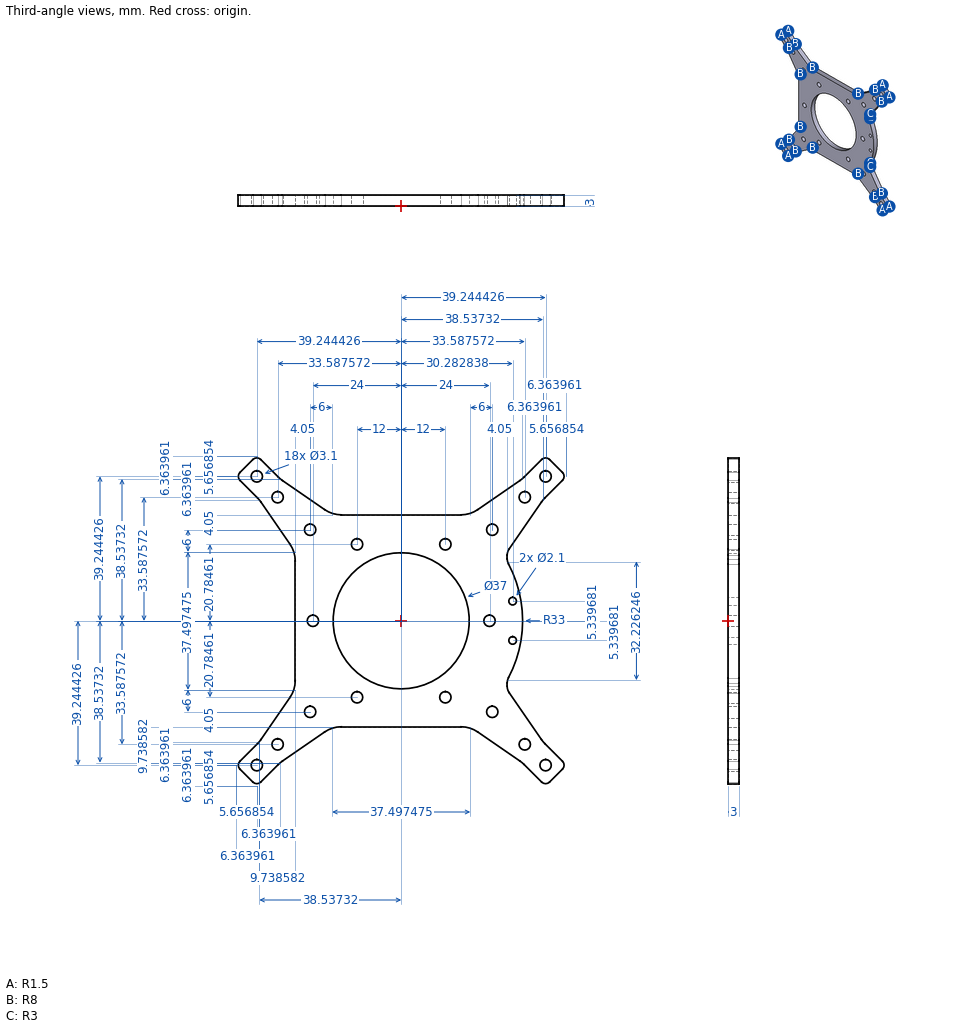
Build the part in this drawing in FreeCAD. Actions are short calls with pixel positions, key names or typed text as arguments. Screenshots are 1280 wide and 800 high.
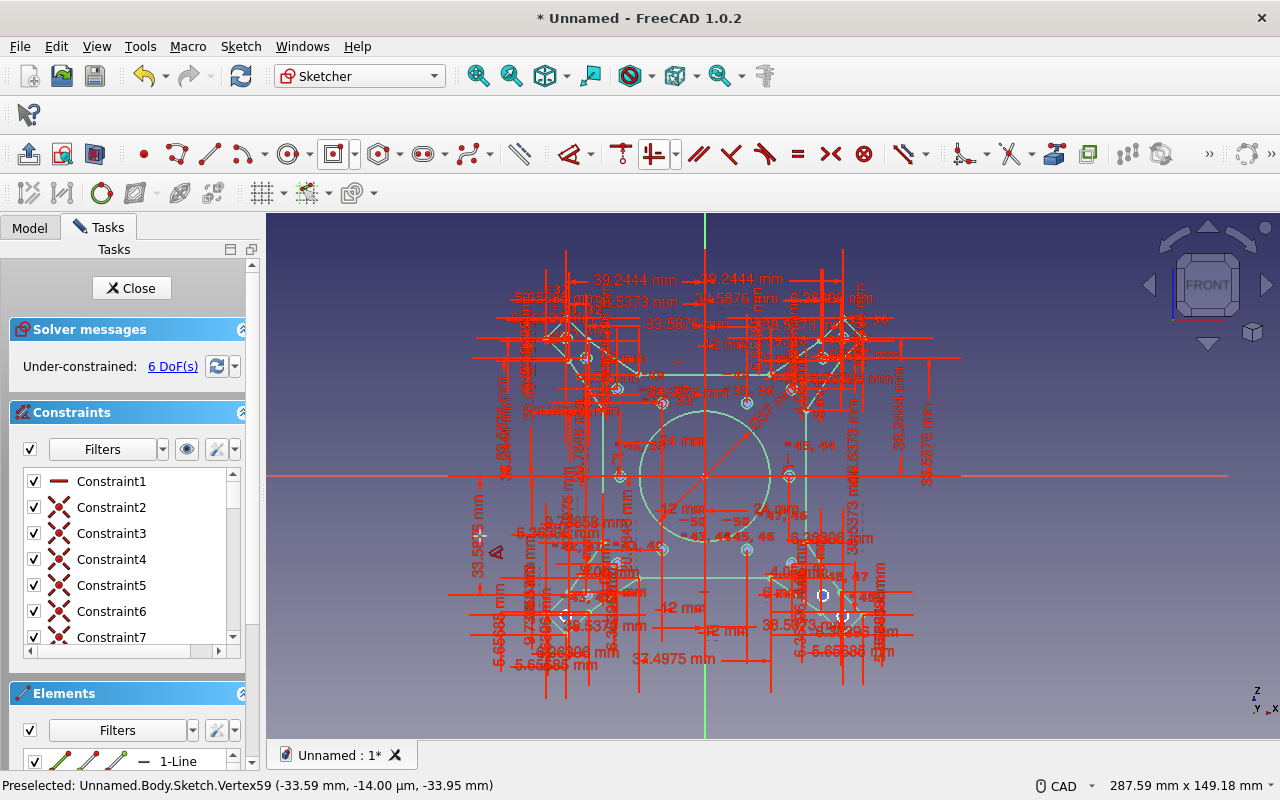
click(566, 616)
click(635, 698)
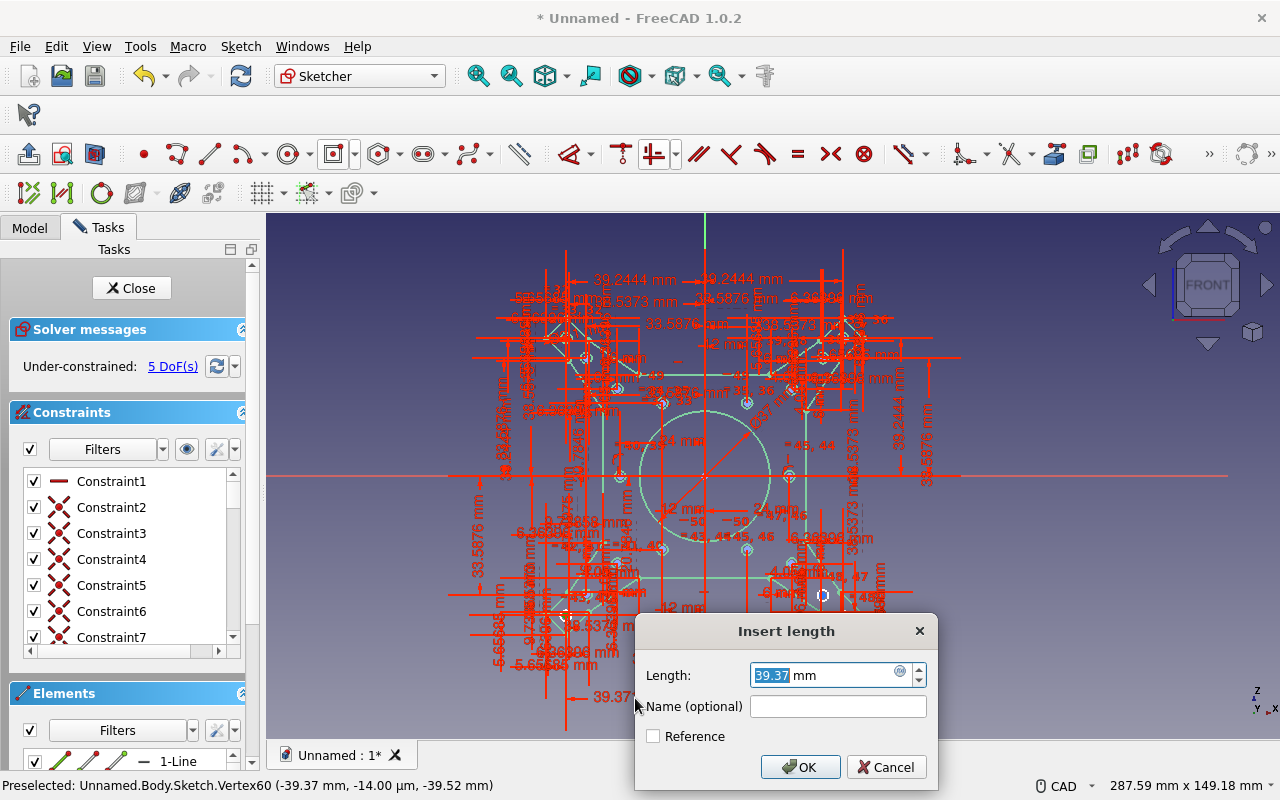
text(39.244426)
key(Return)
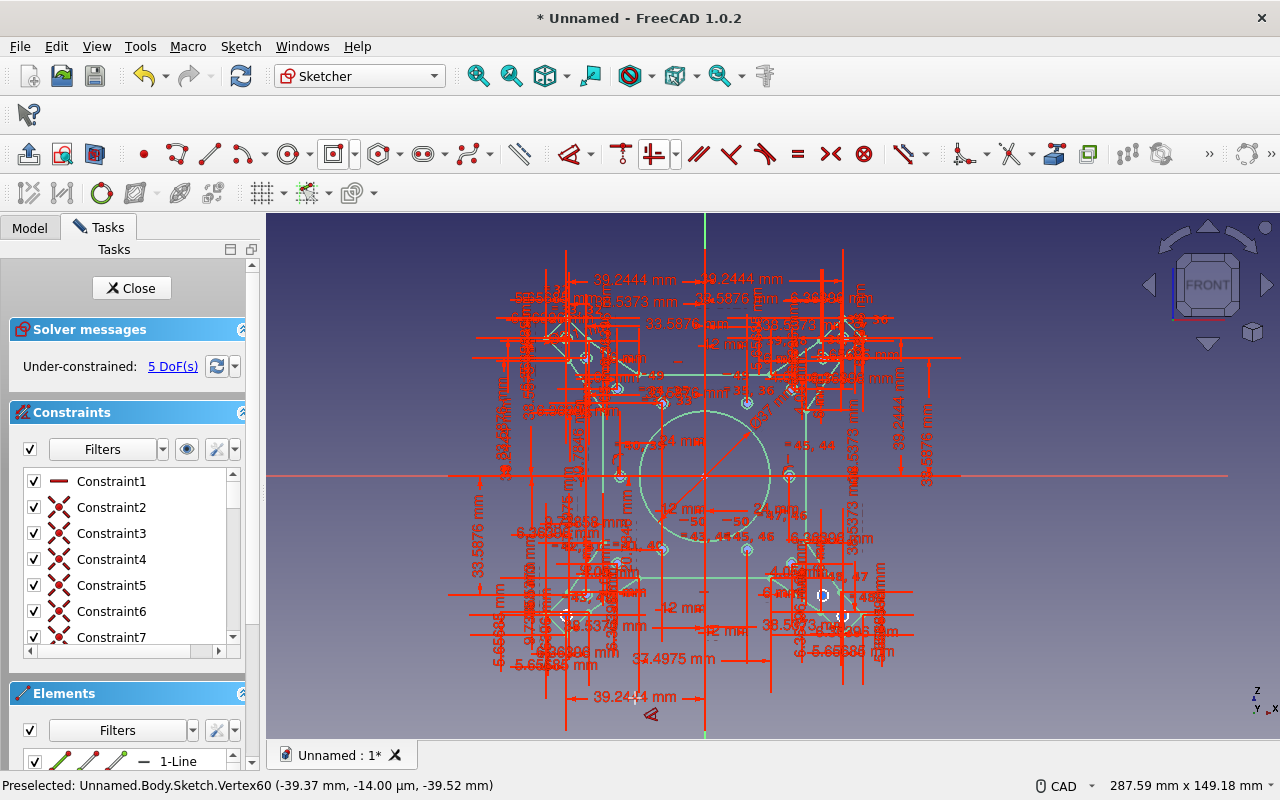
click(566, 616)
click(484, 514)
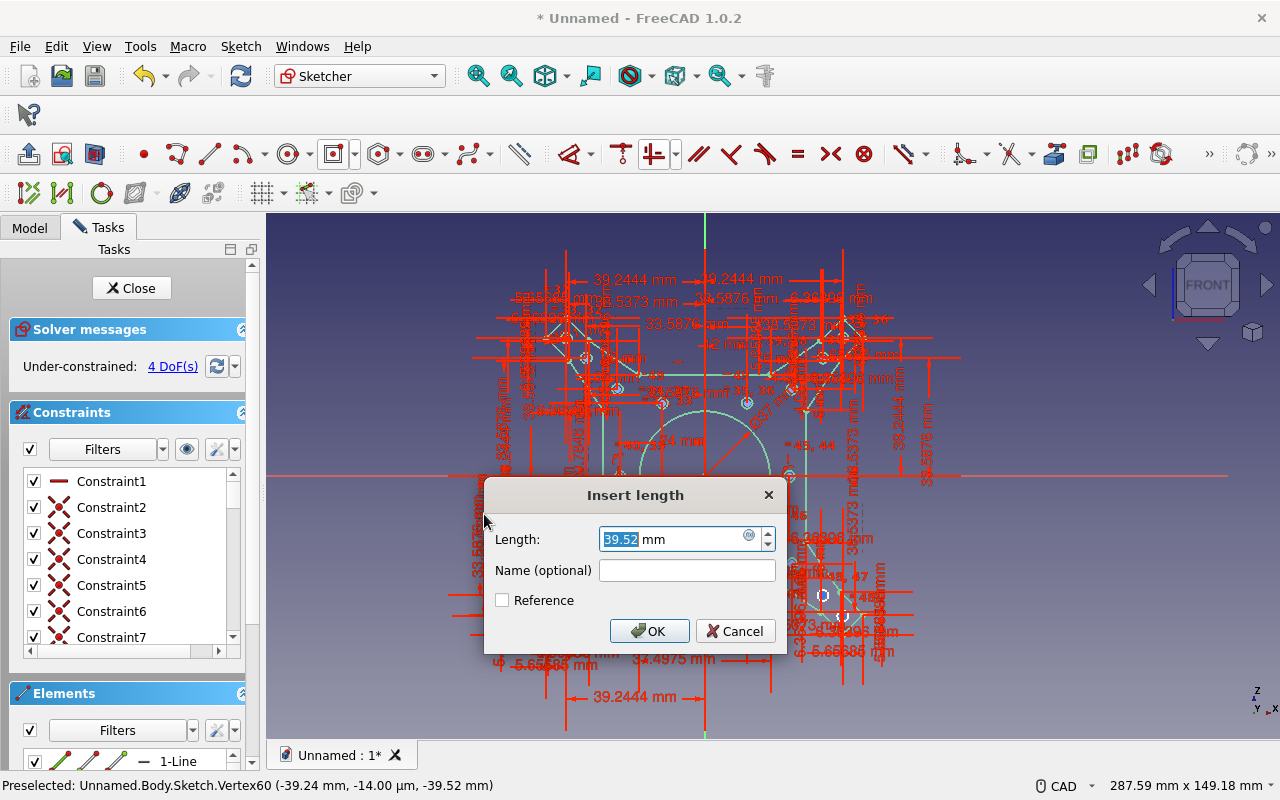
text(39.244426)
key(Return)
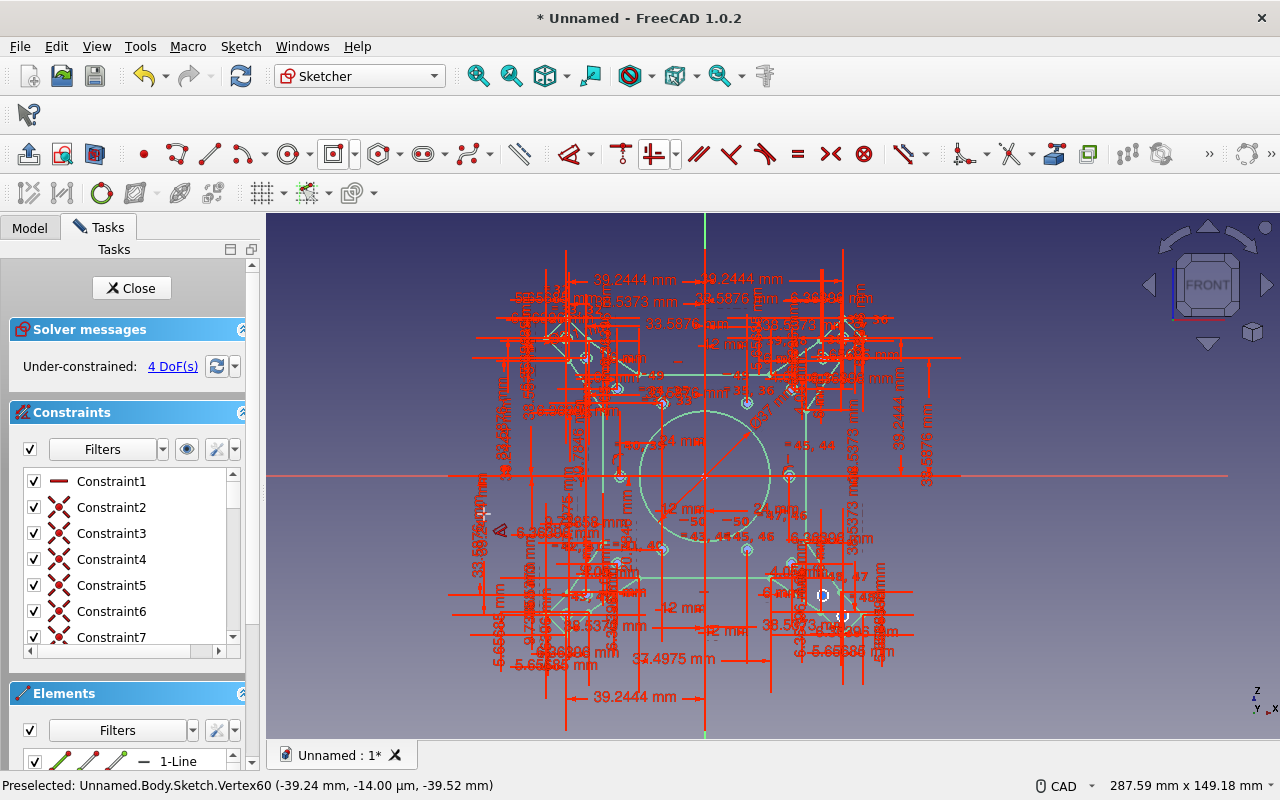
click(823, 596)
click(764, 654)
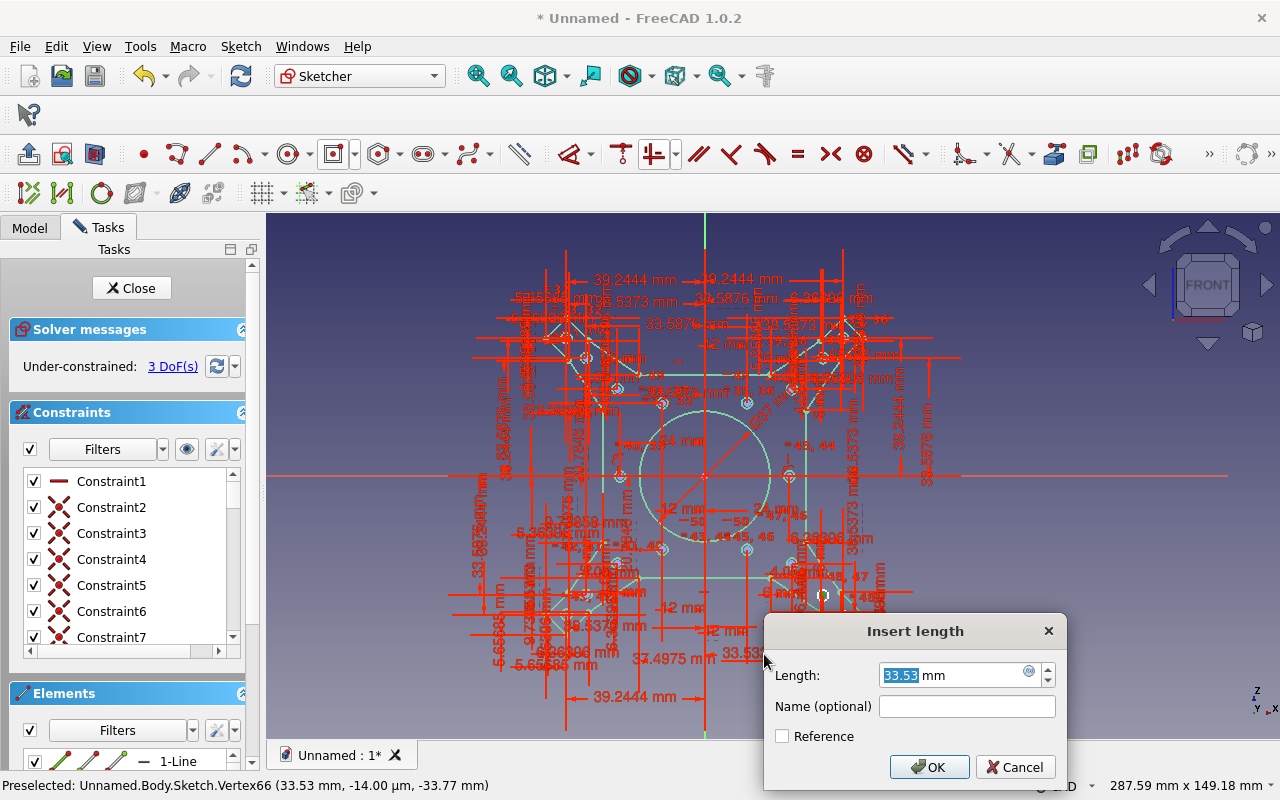
text(33.587572)
key(Return)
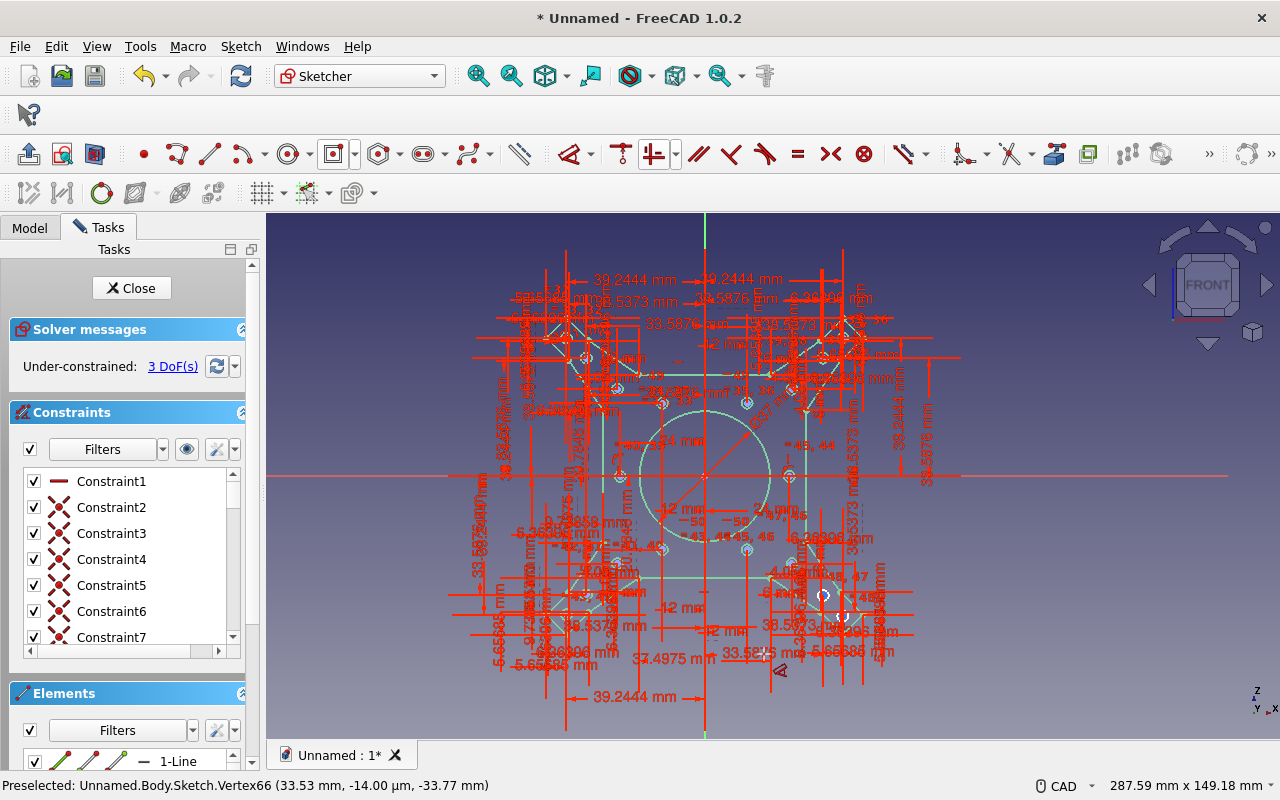
click(823, 596)
click(881, 578)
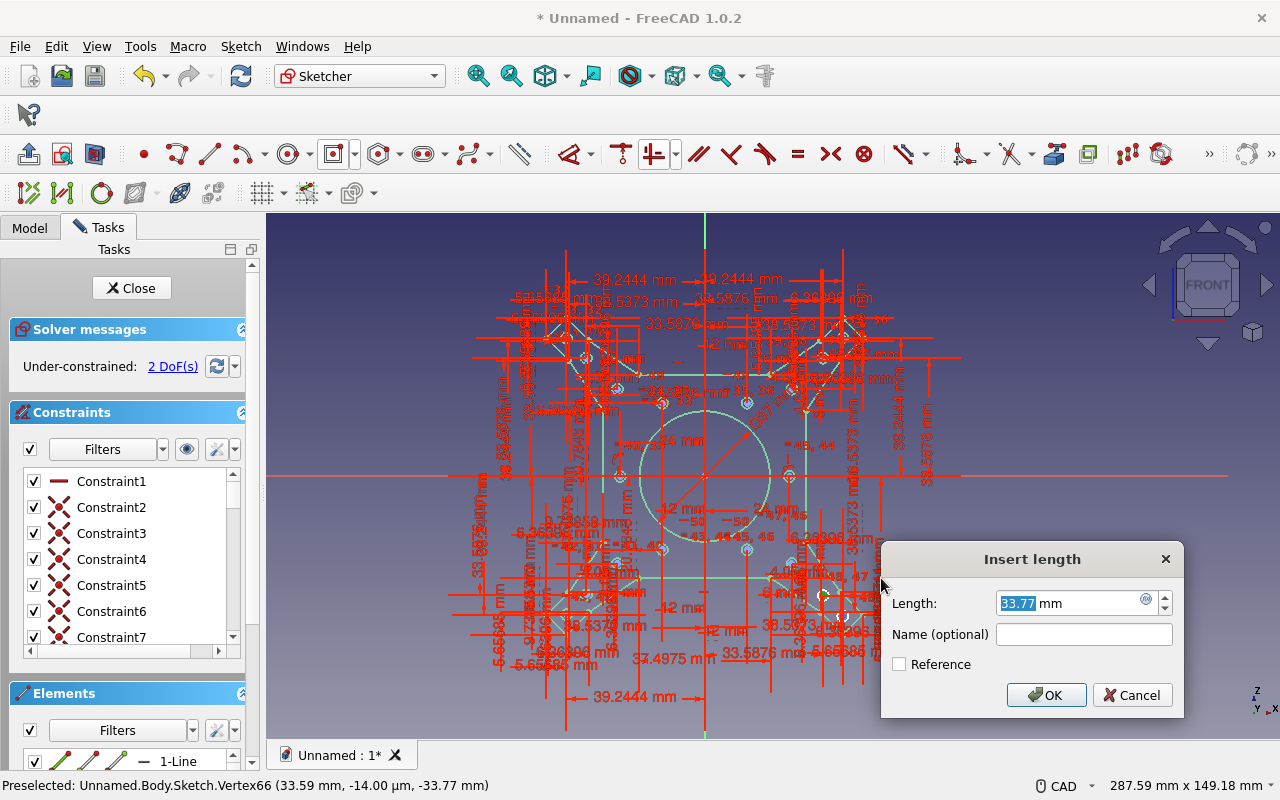
text(33.587572)
key(Return)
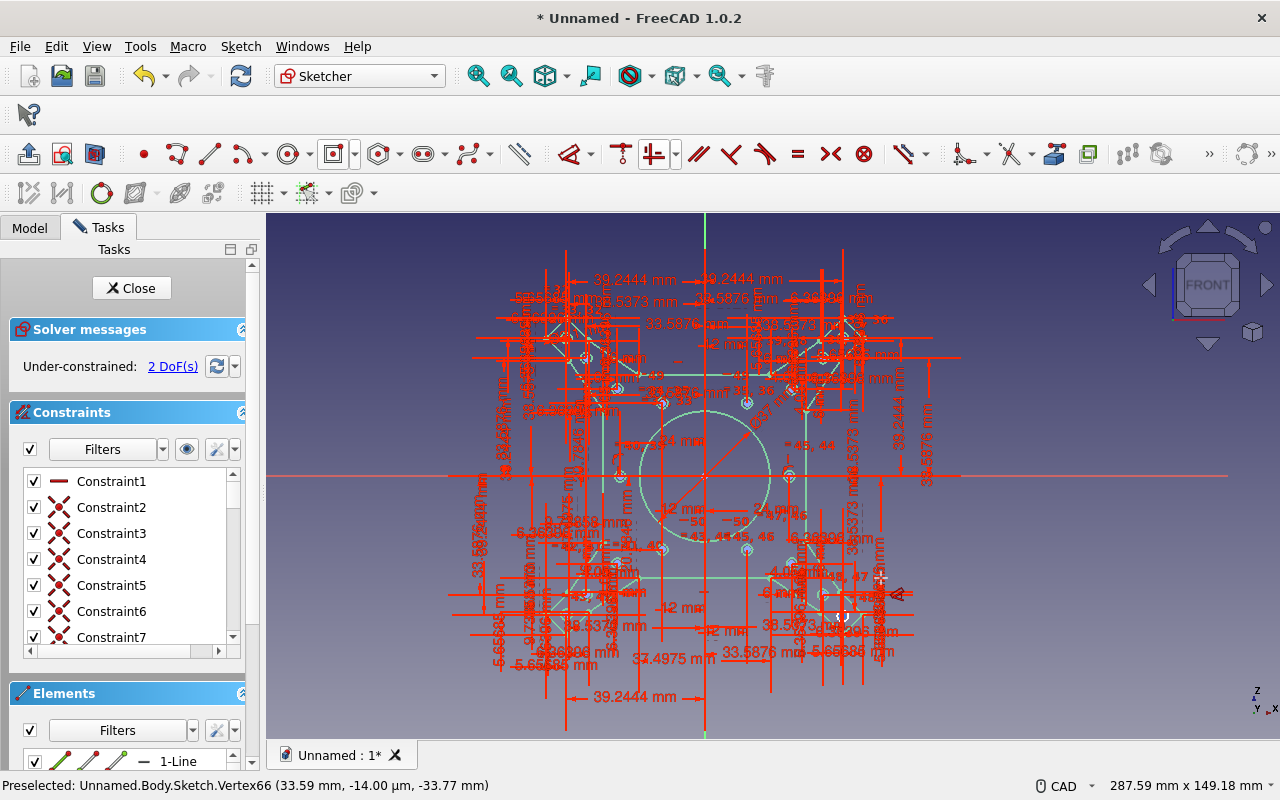
click(843, 616)
click(774, 674)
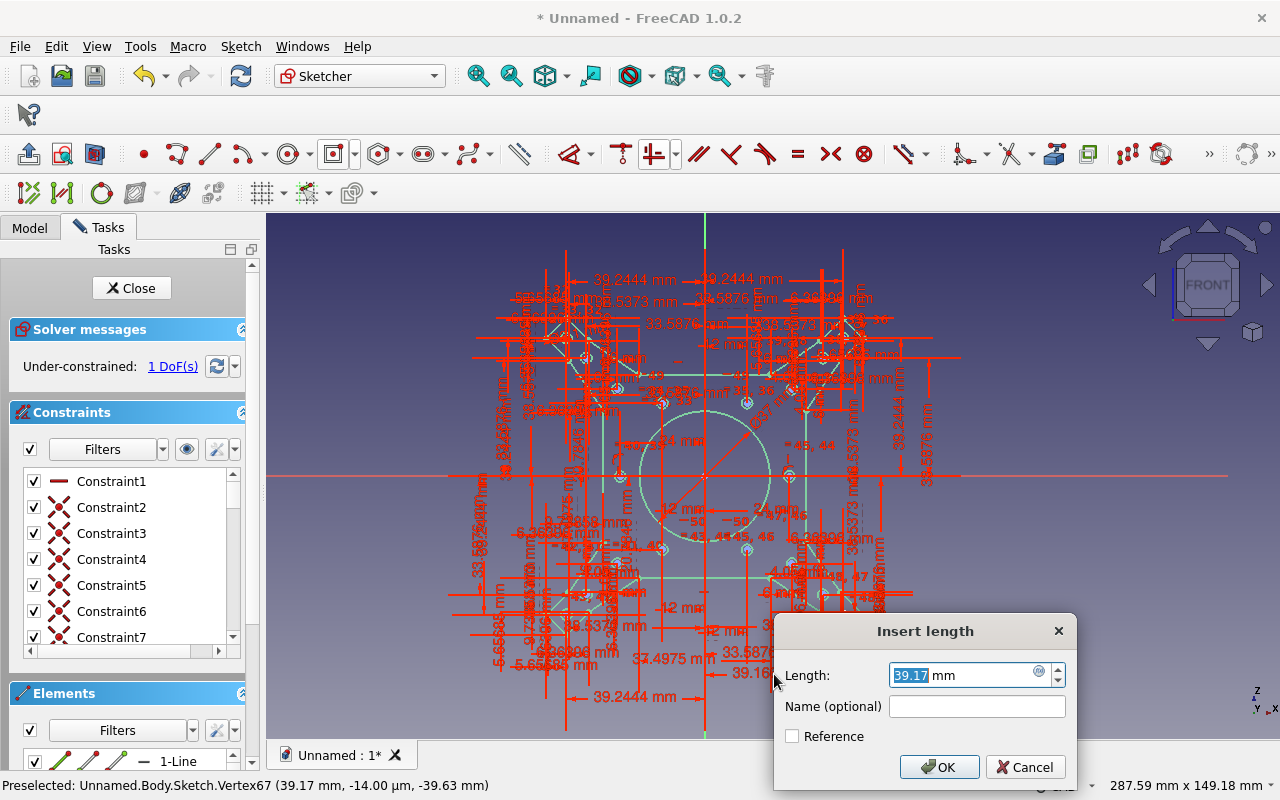
text(39.244426)
key(Return)